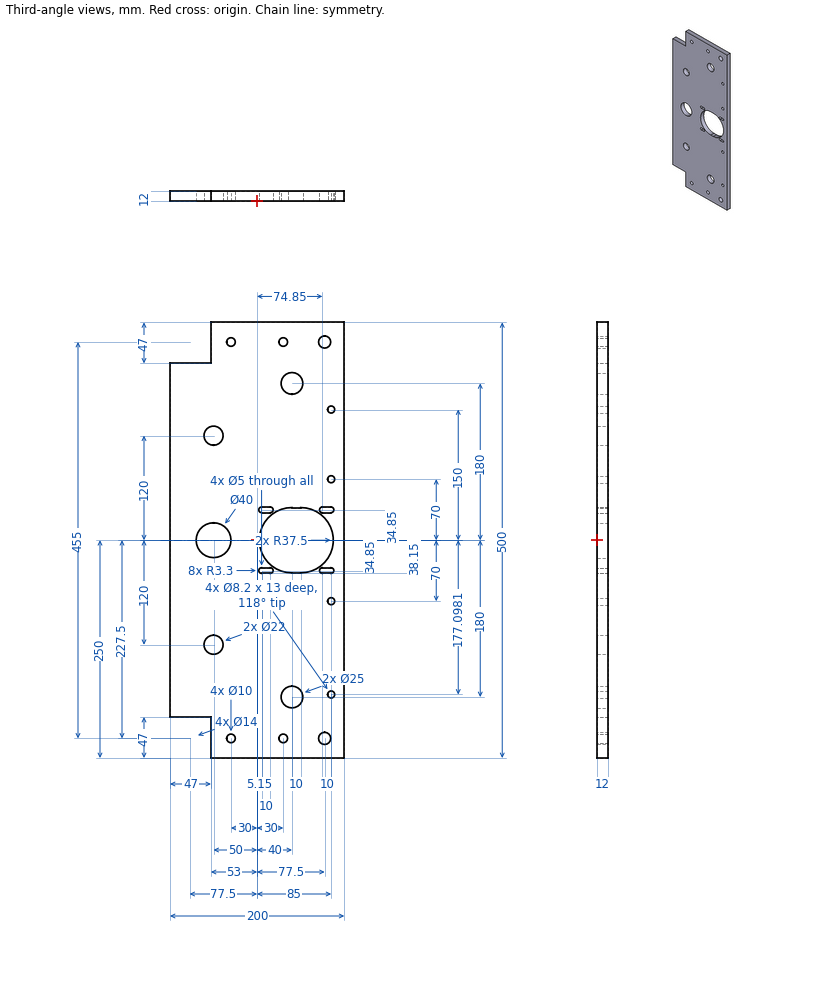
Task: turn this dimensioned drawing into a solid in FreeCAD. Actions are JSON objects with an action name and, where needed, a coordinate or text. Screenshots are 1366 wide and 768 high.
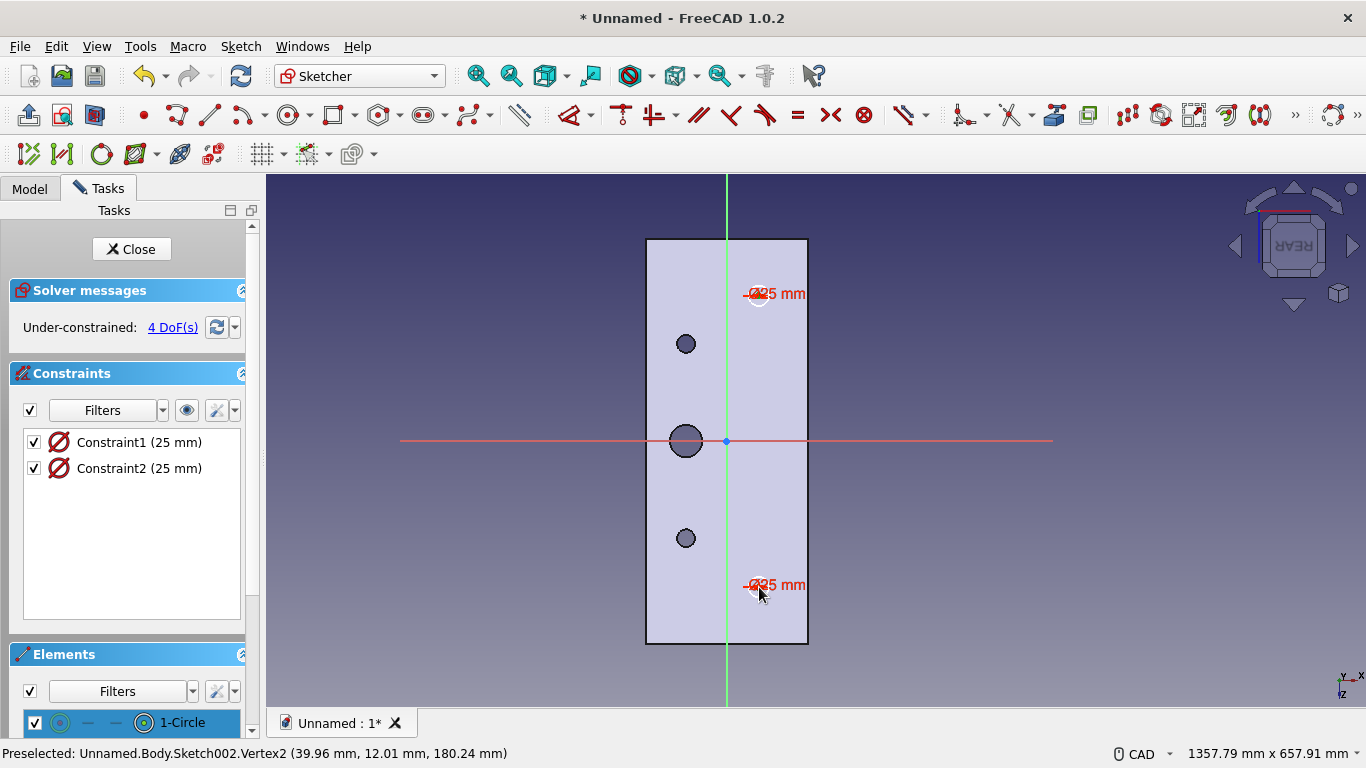
{"action": "key", "text": "v"}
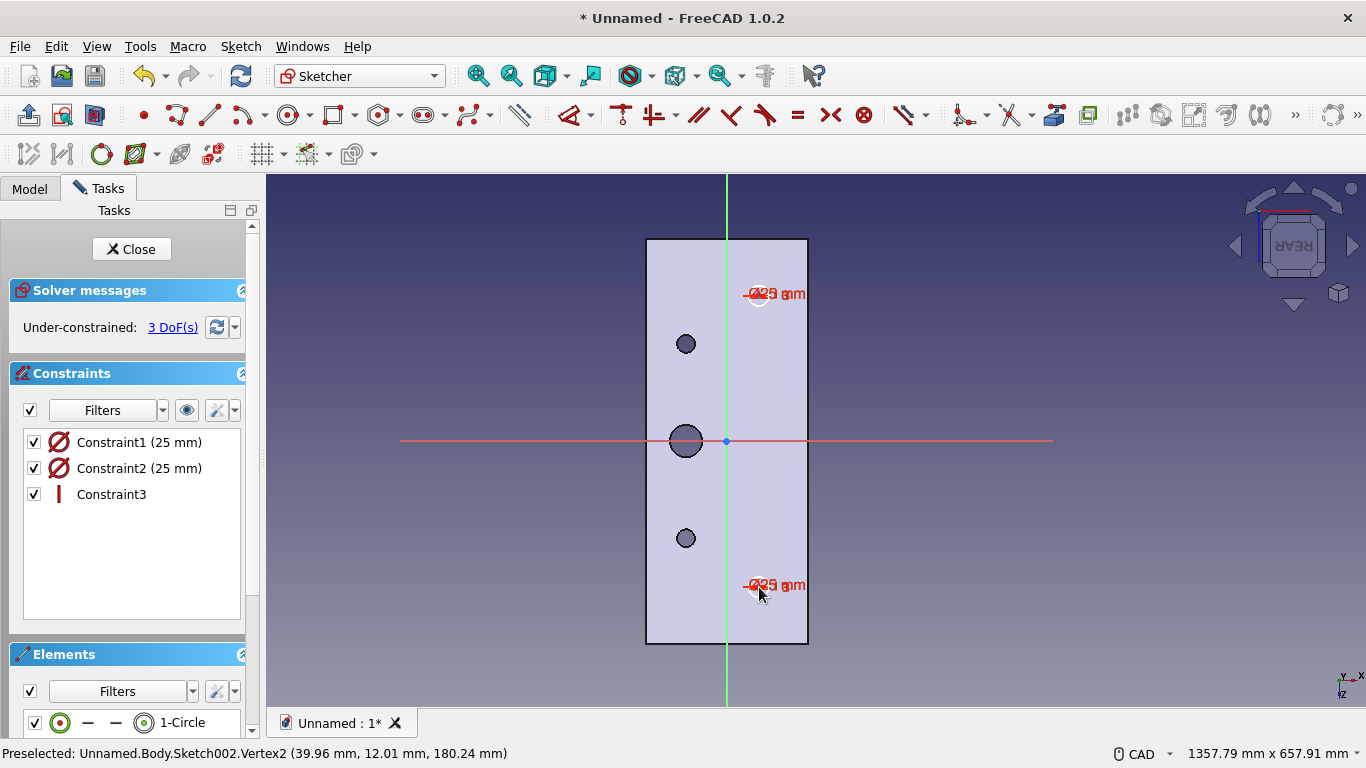
{"action": "key", "text": "d"}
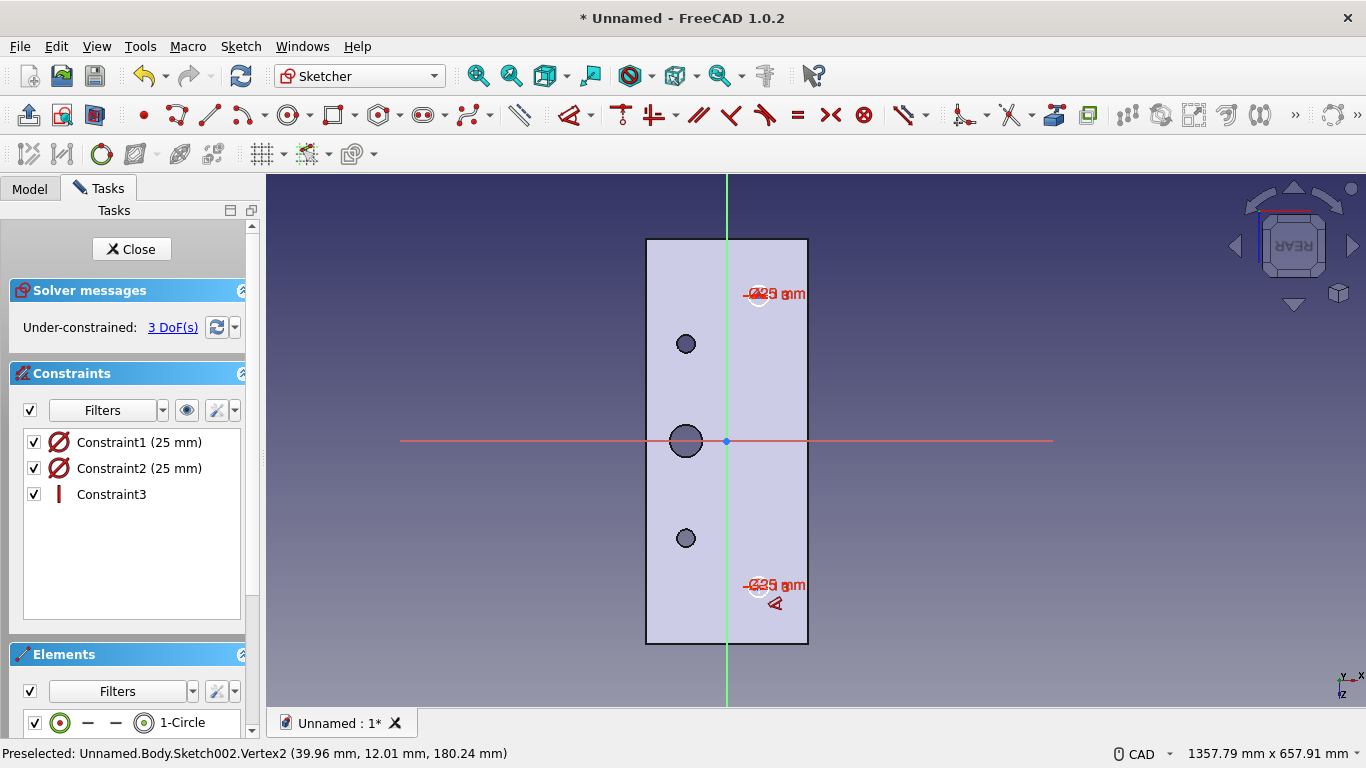
{"action": "scroll", "coordinate": [759, 296], "scroll_direction": "up", "scroll_amount": 2}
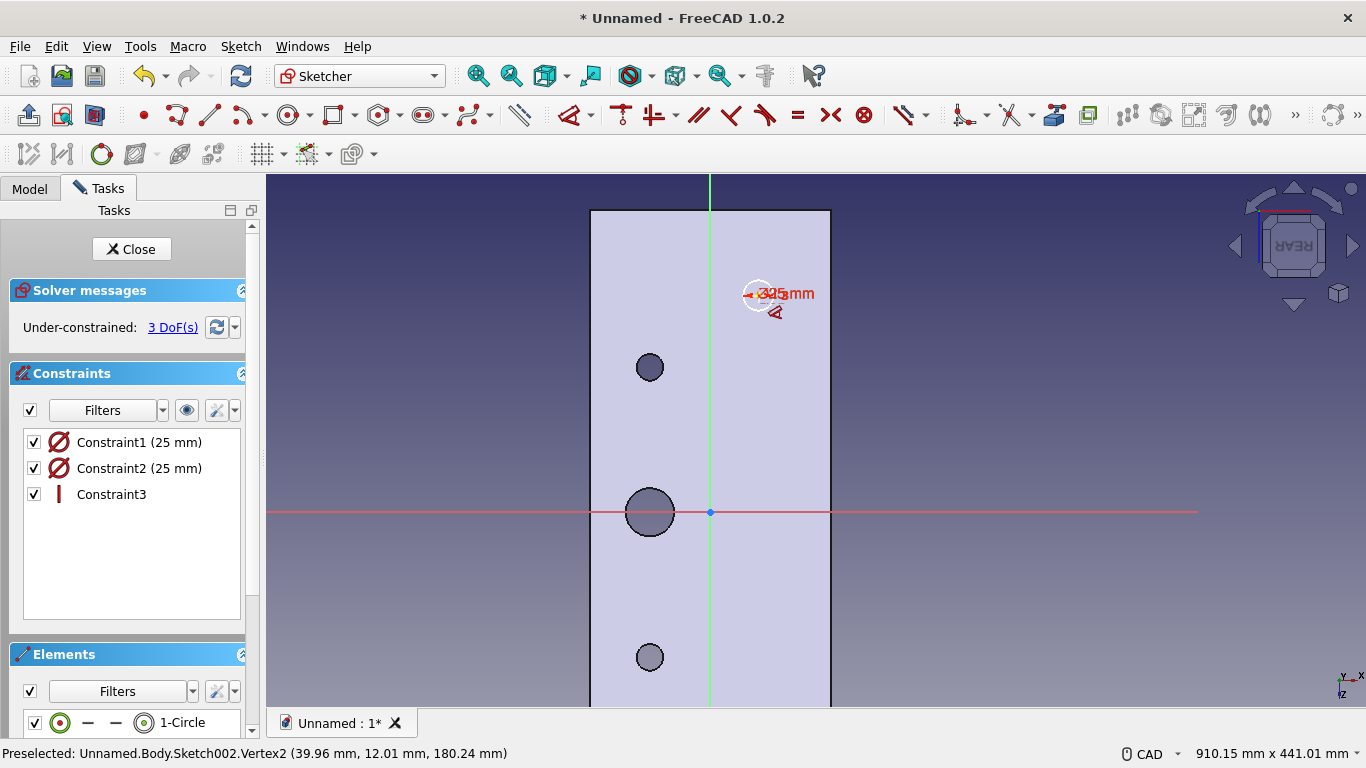
{"action": "left_click", "coordinate": [758, 296]}
{"action": "left_click", "coordinate": [734, 262]}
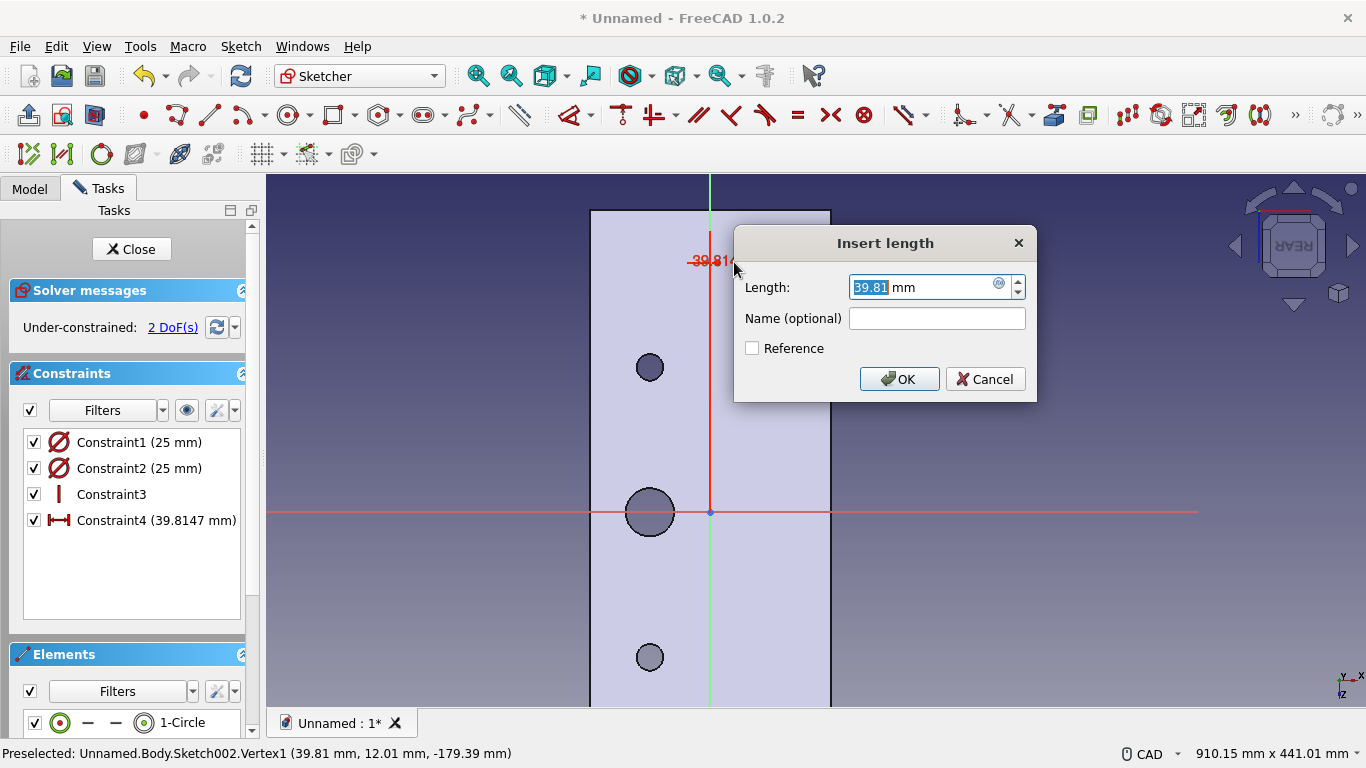
{"action": "type", "text": "40"}
{"action": "key", "text": "Return"}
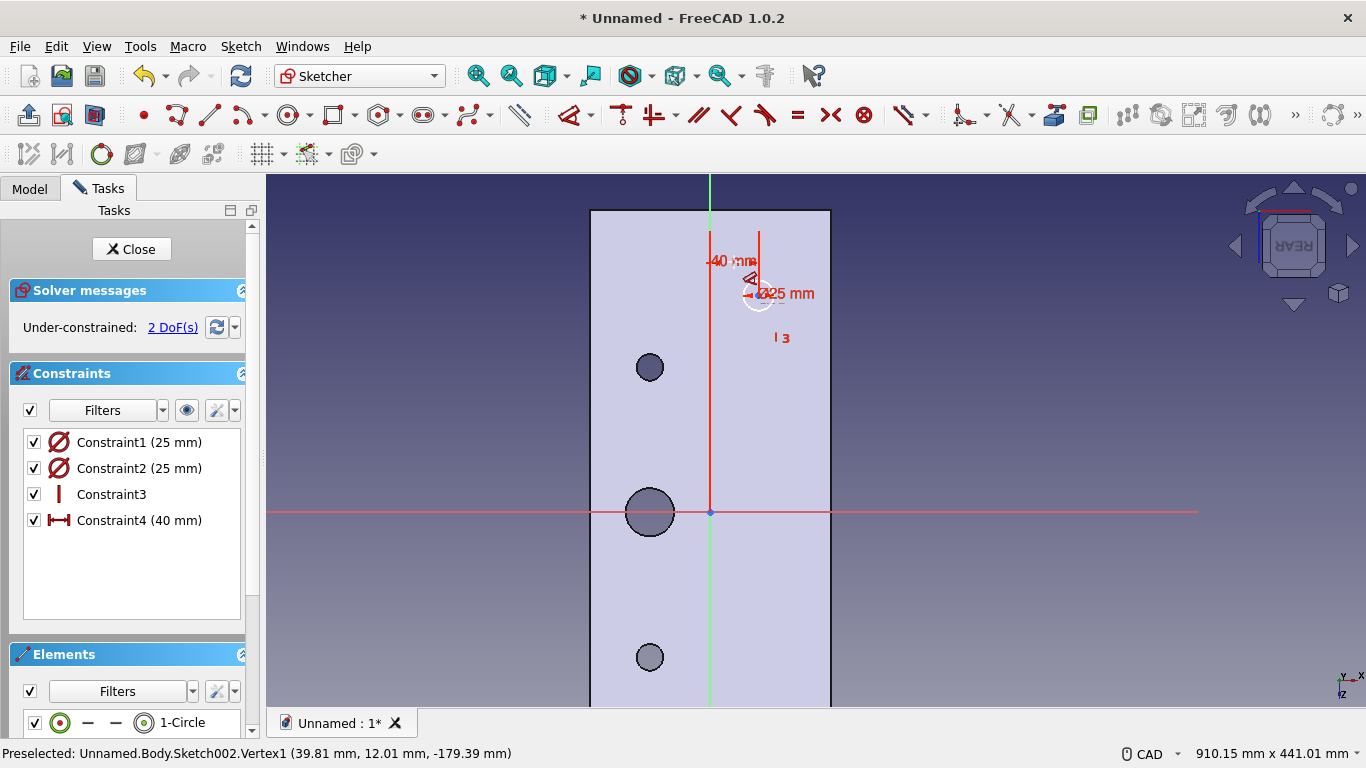
{"action": "left_click", "coordinate": [759, 296]}
{"action": "left_click", "coordinate": [676, 404]}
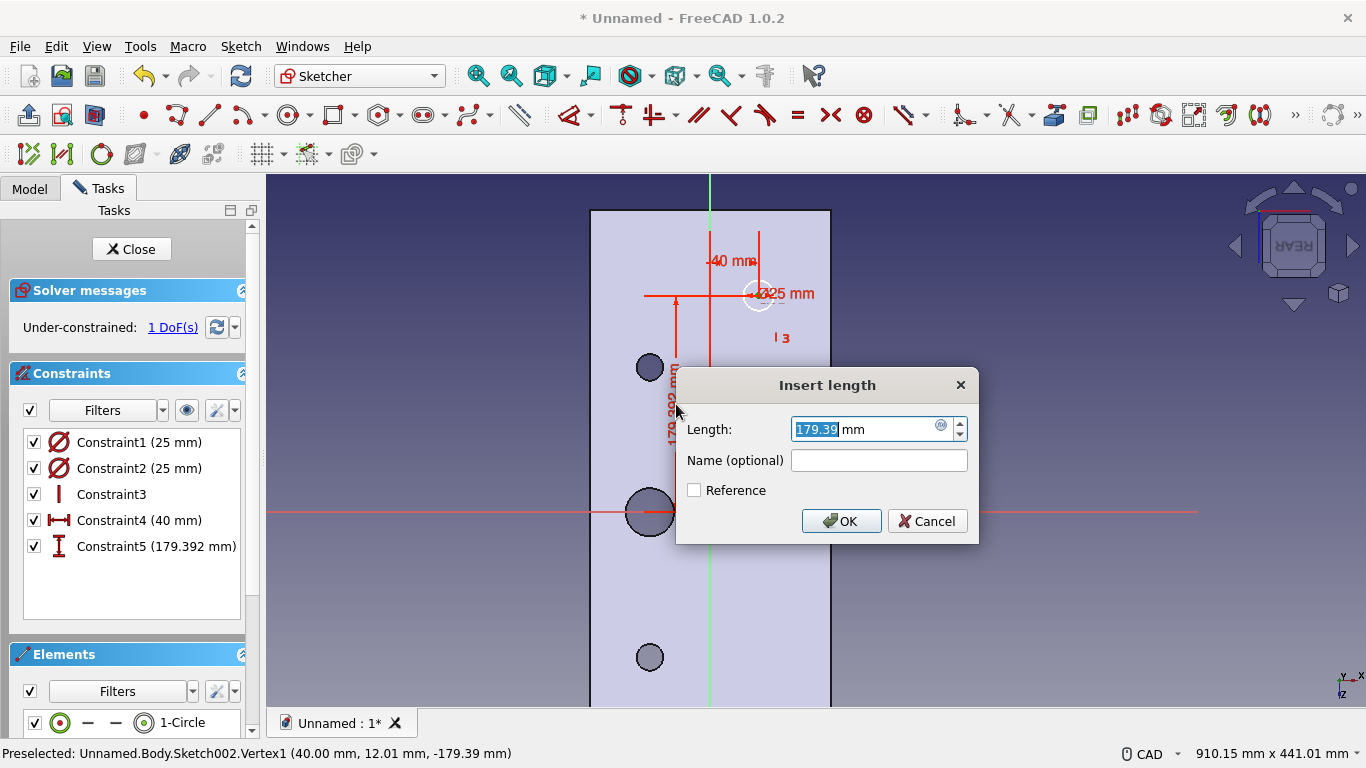
{"action": "type", "text": "180"}
{"action": "key", "text": "Return"}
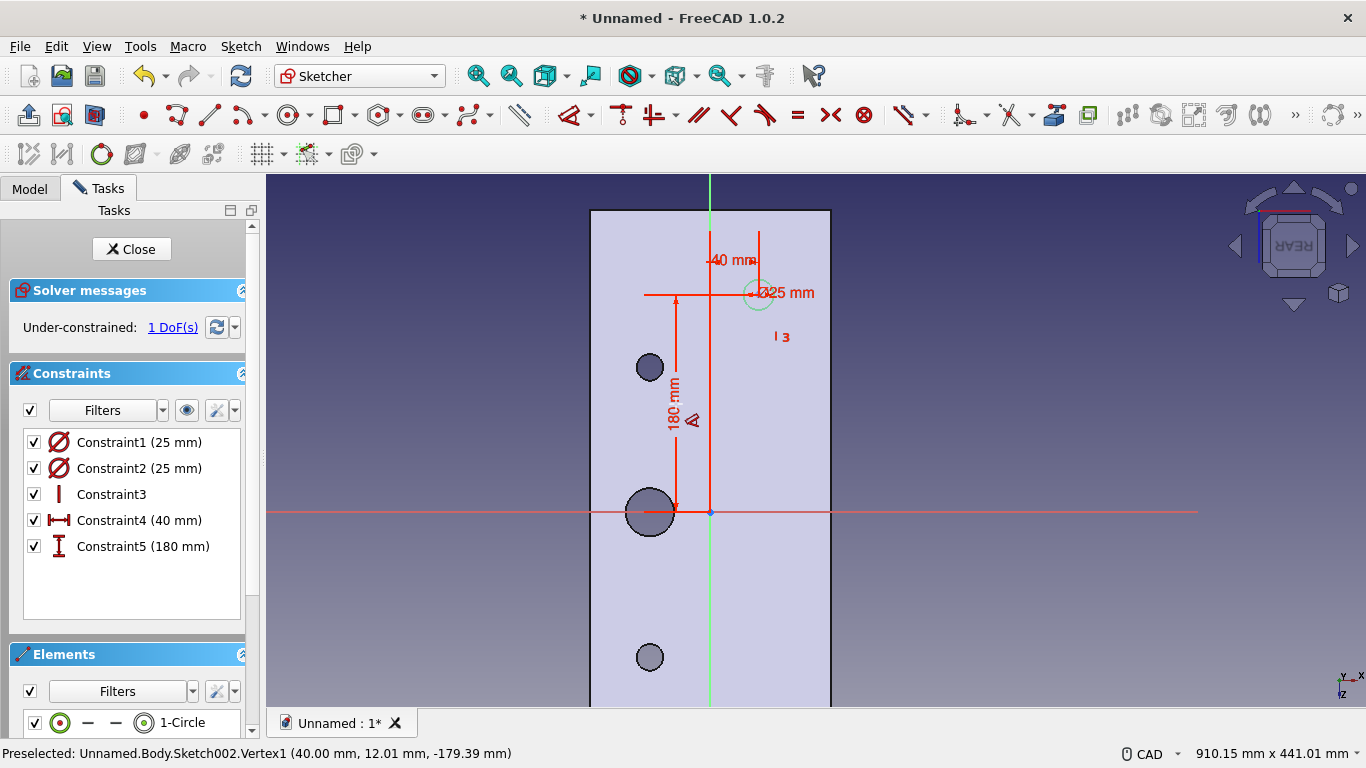
{"action": "scroll", "coordinate": [759, 294], "scroll_direction": "down", "scroll_amount": 2}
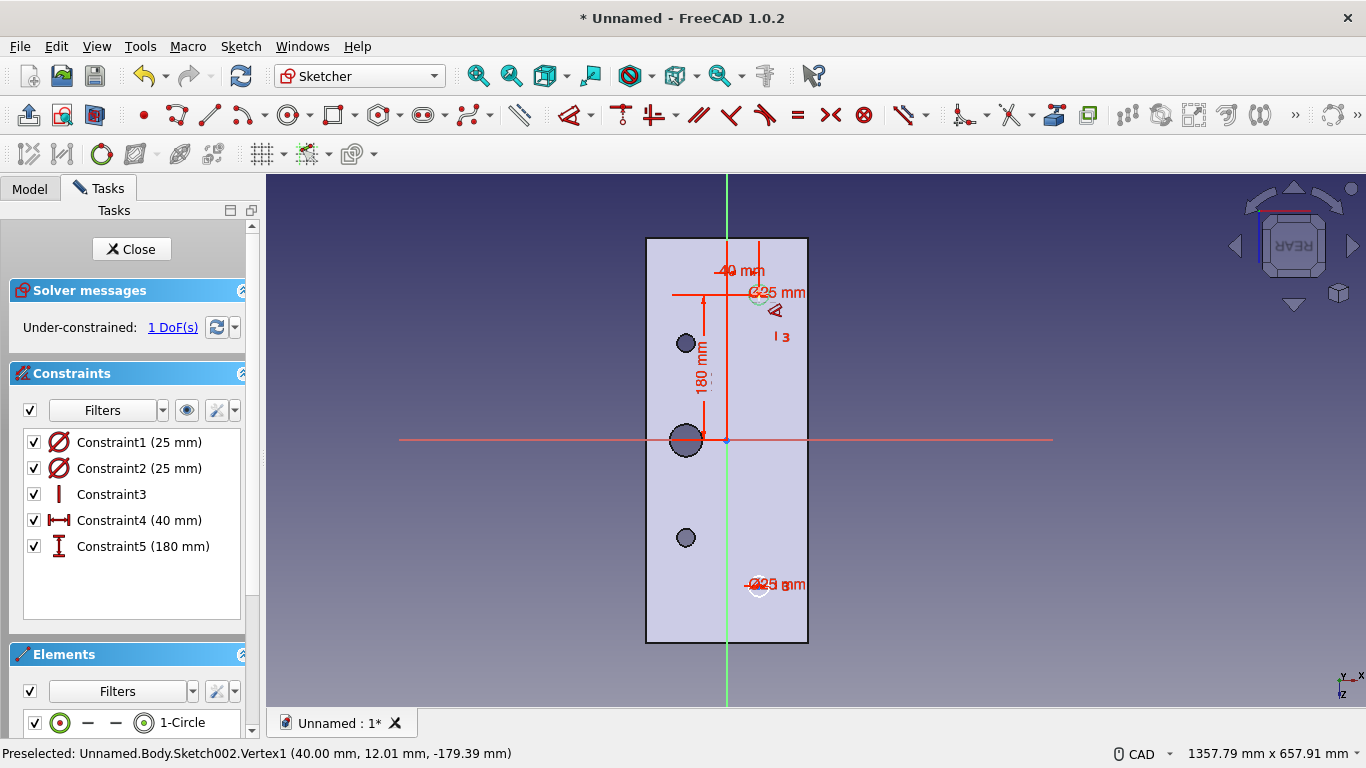
{"action": "left_click", "coordinate": [759, 586]}
{"action": "left_click", "coordinate": [693, 513]}